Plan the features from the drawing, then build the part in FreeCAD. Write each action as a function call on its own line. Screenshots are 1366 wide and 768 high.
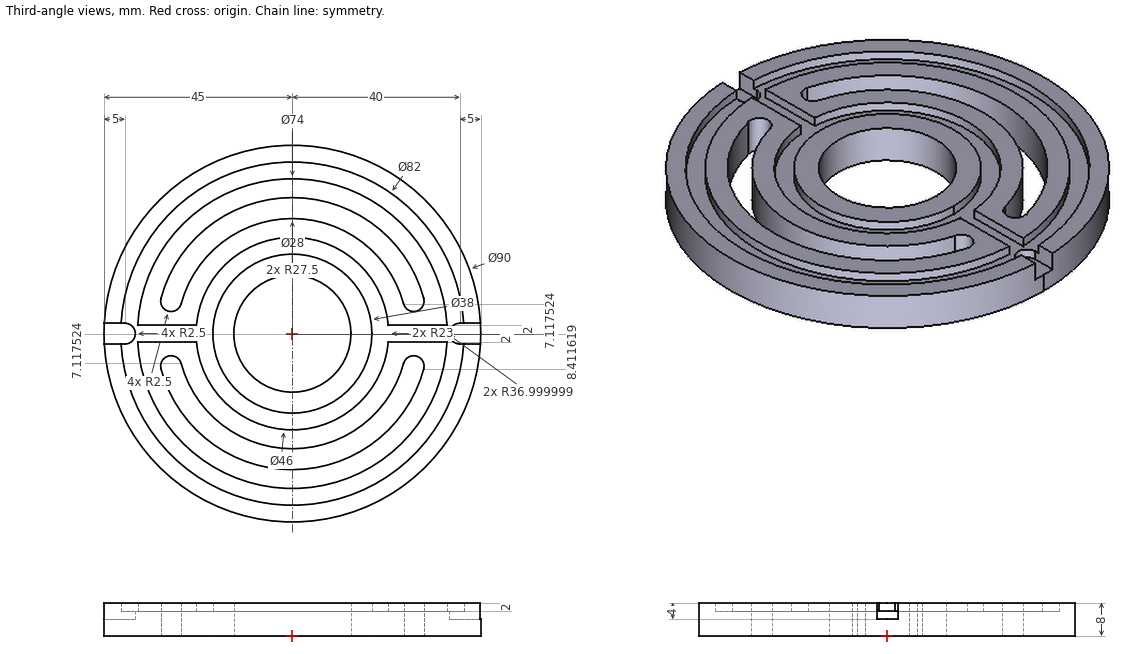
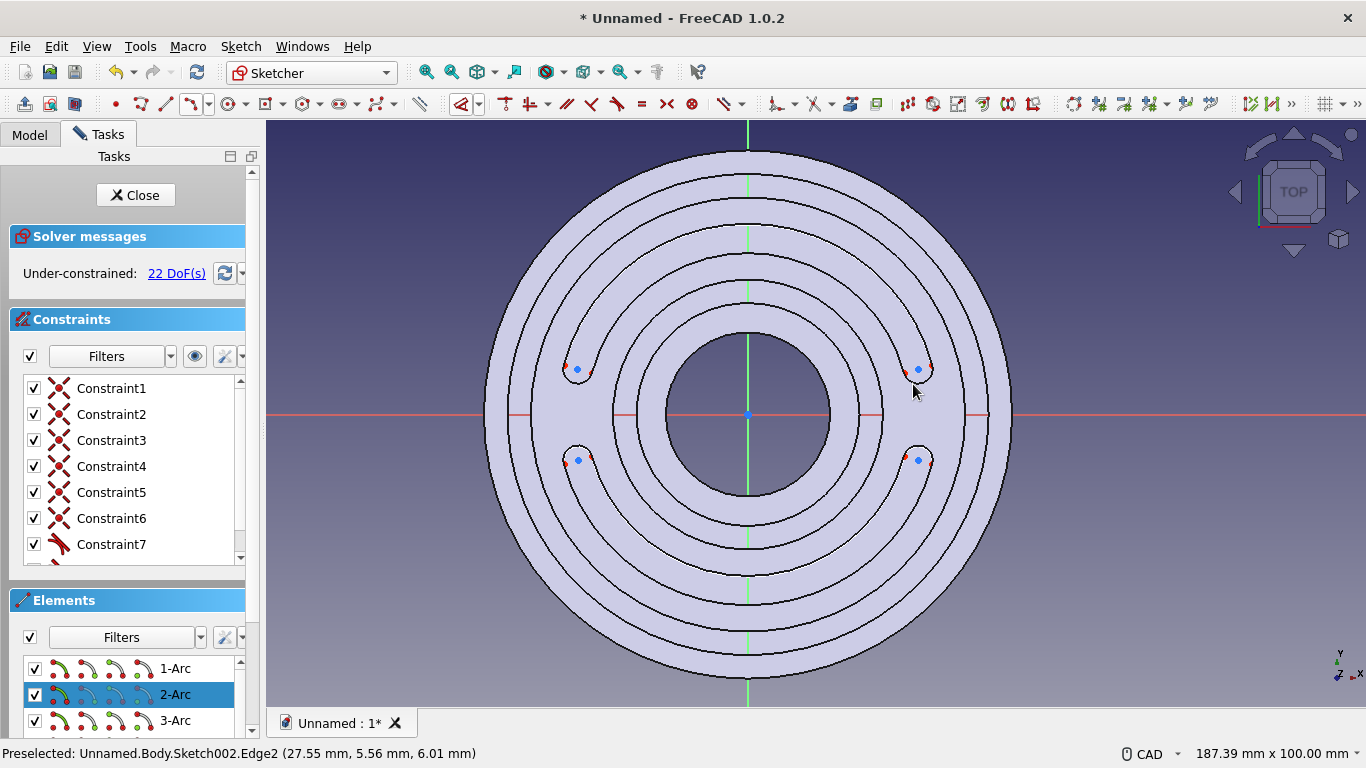
click(843, 250)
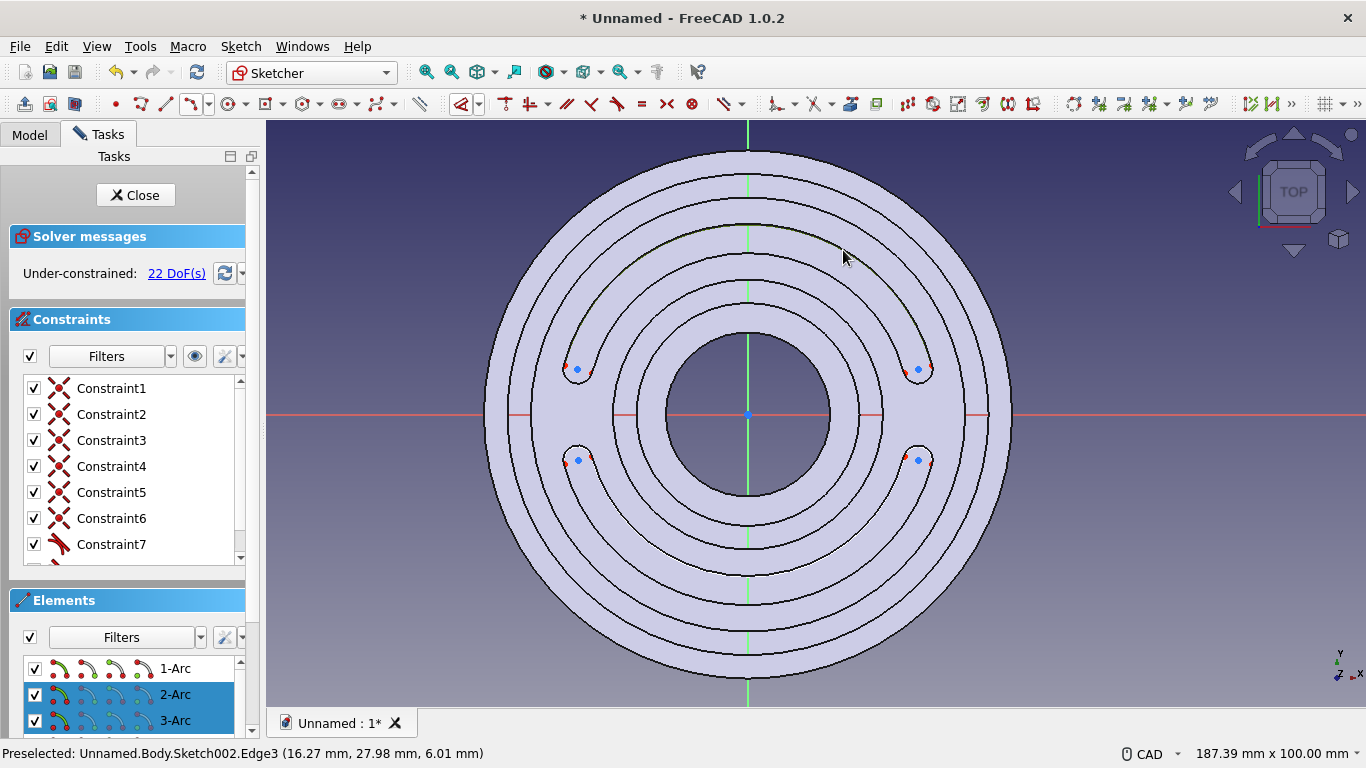
click(617, 104)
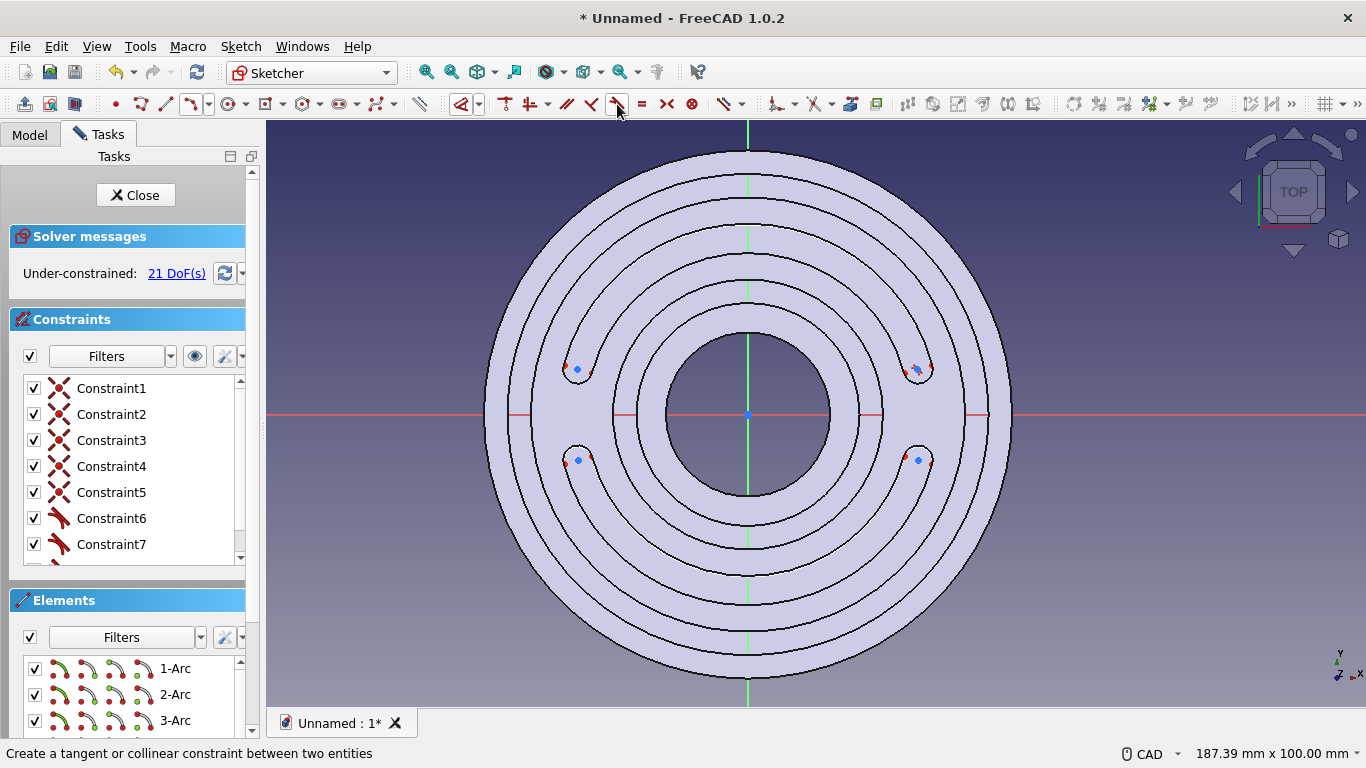
click(843, 250)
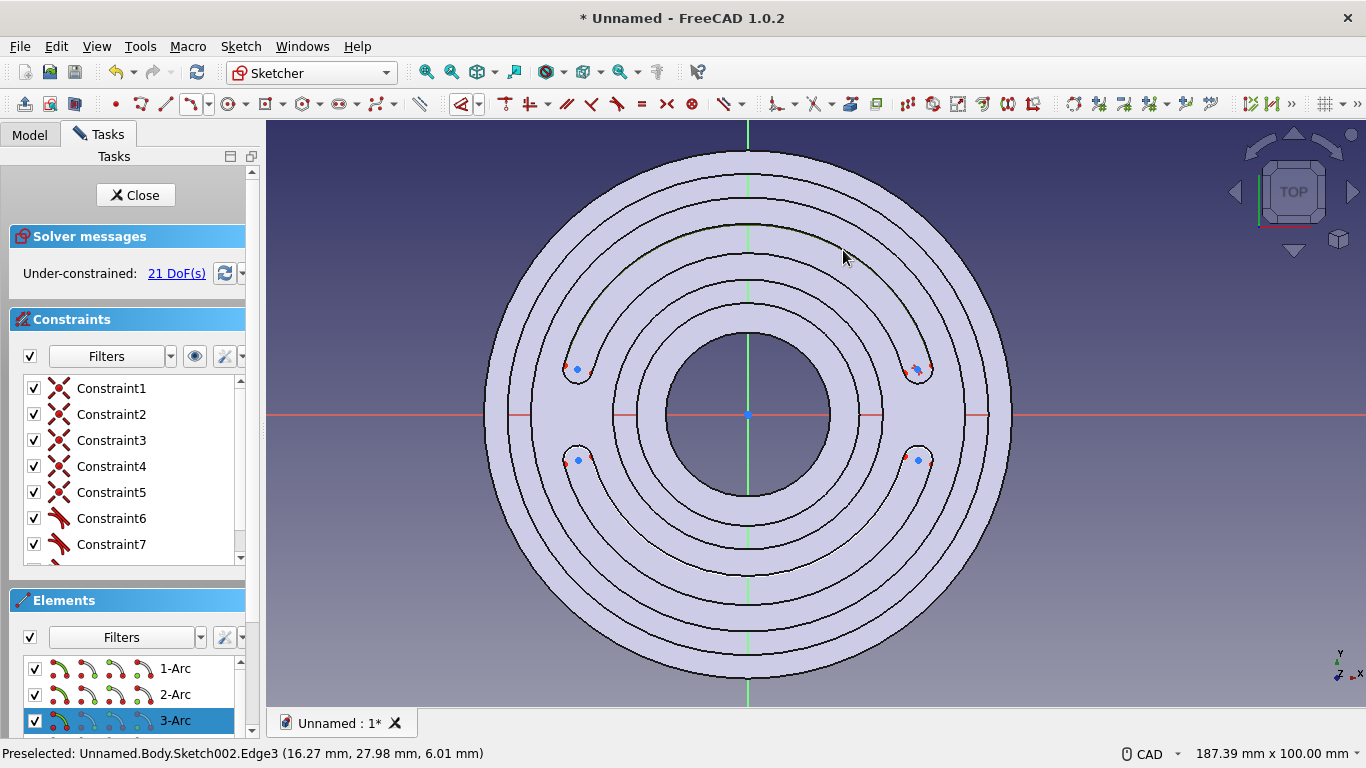
click(567, 379)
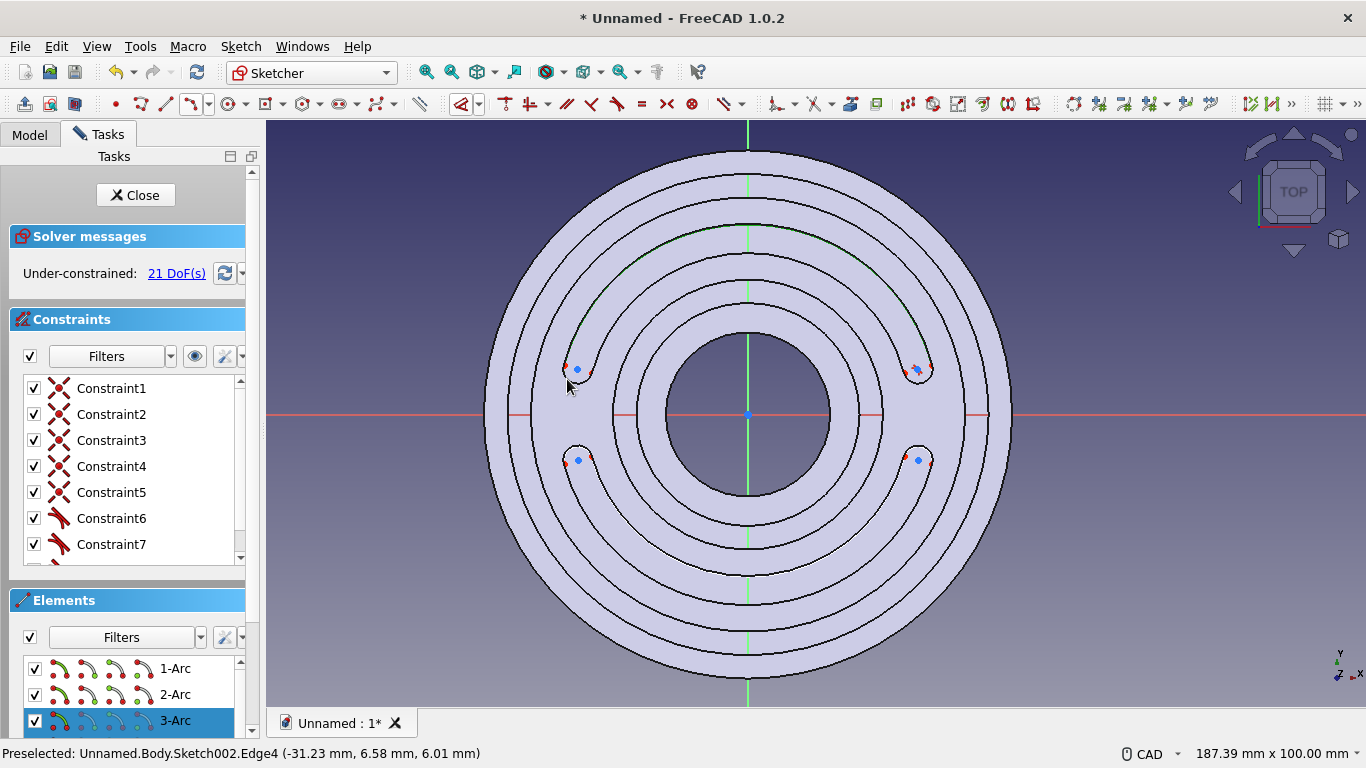
click(617, 104)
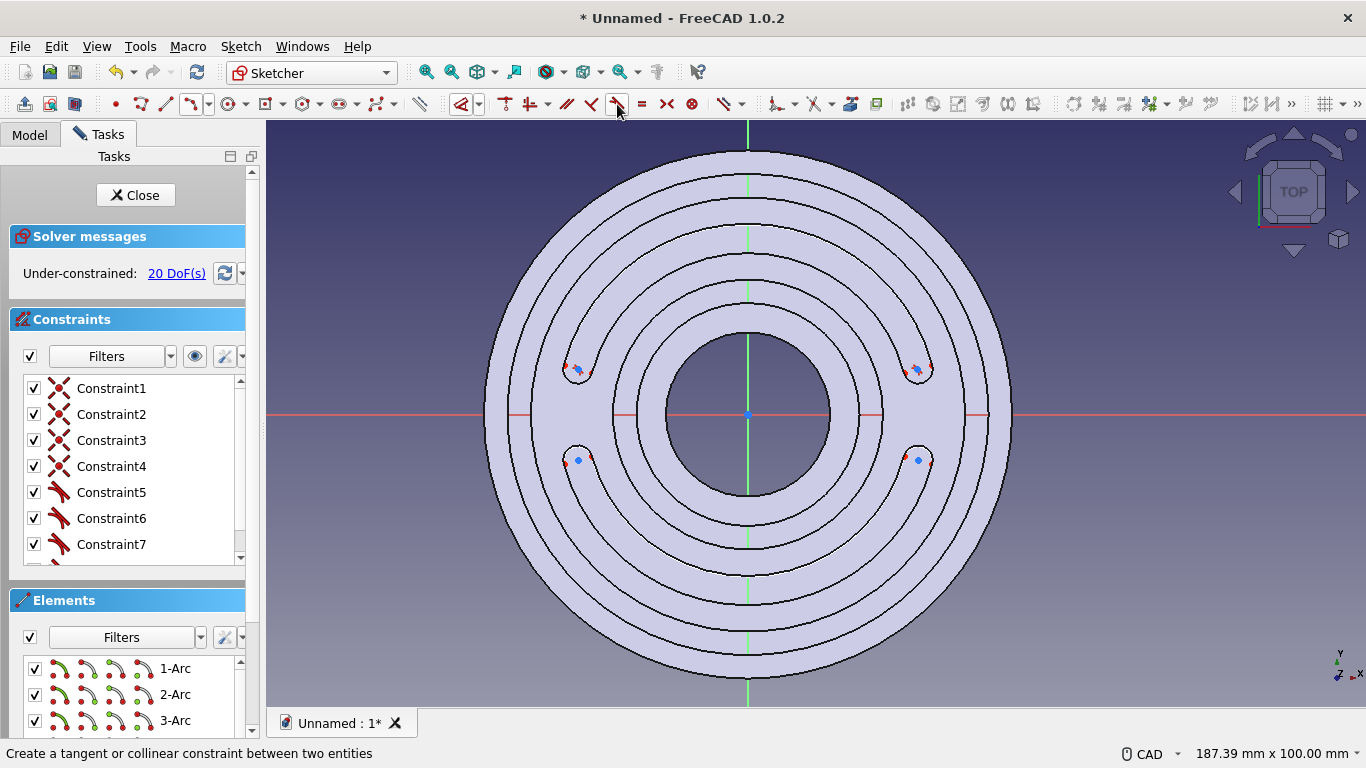
click(583, 447)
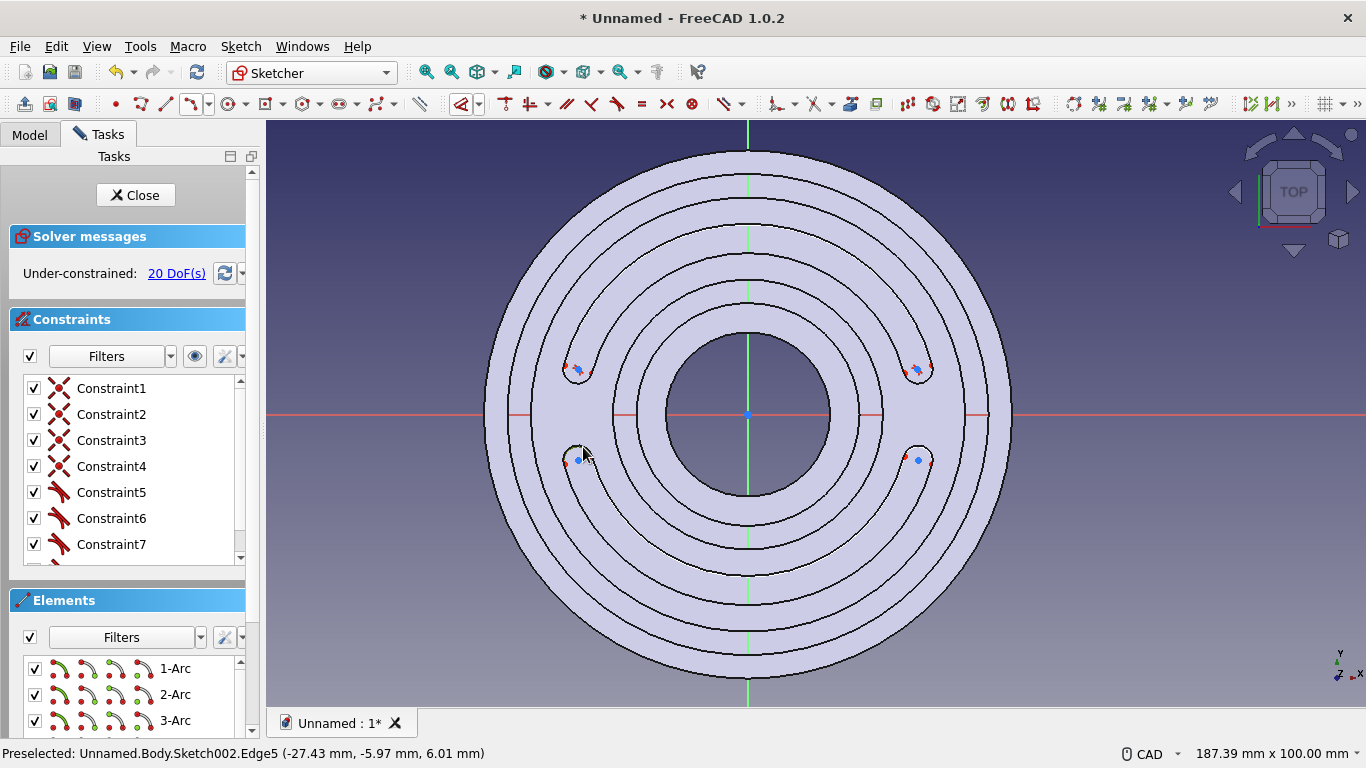
click(653, 581)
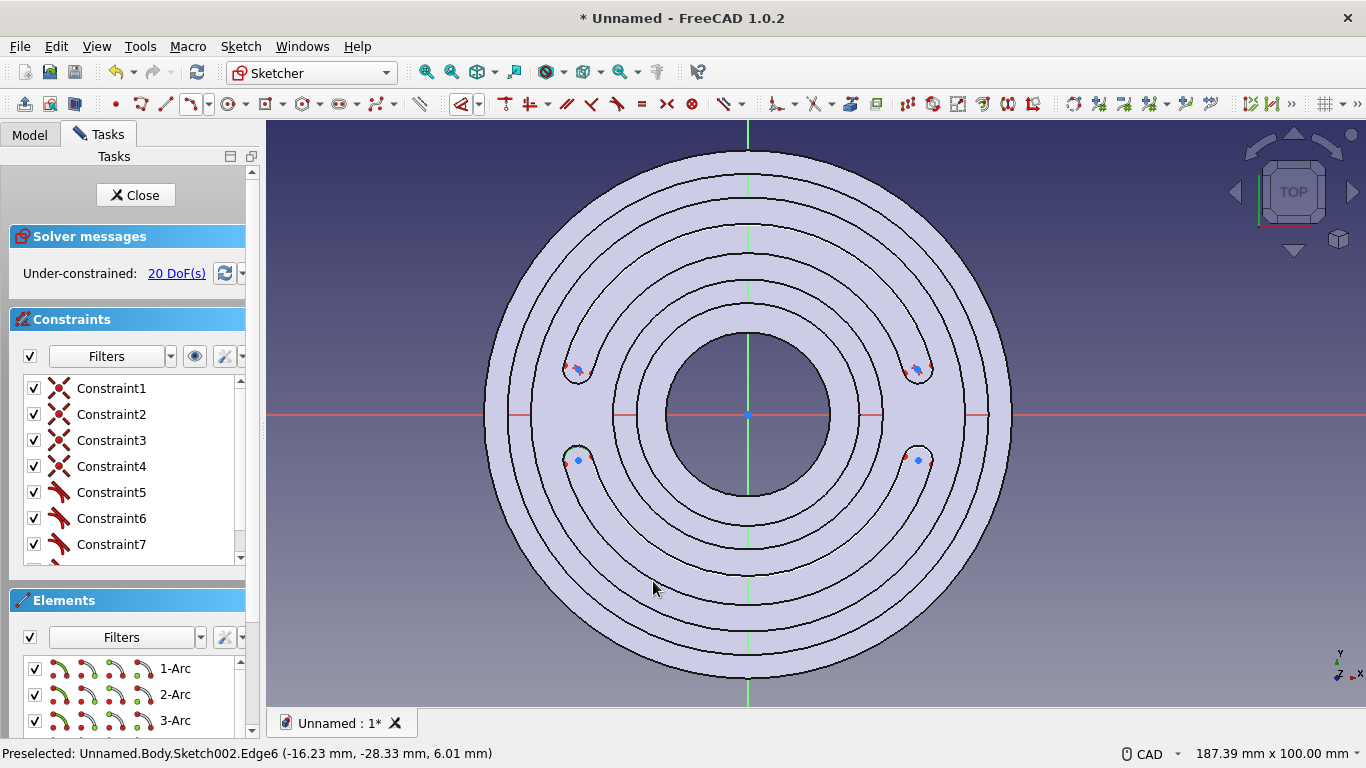
key(t)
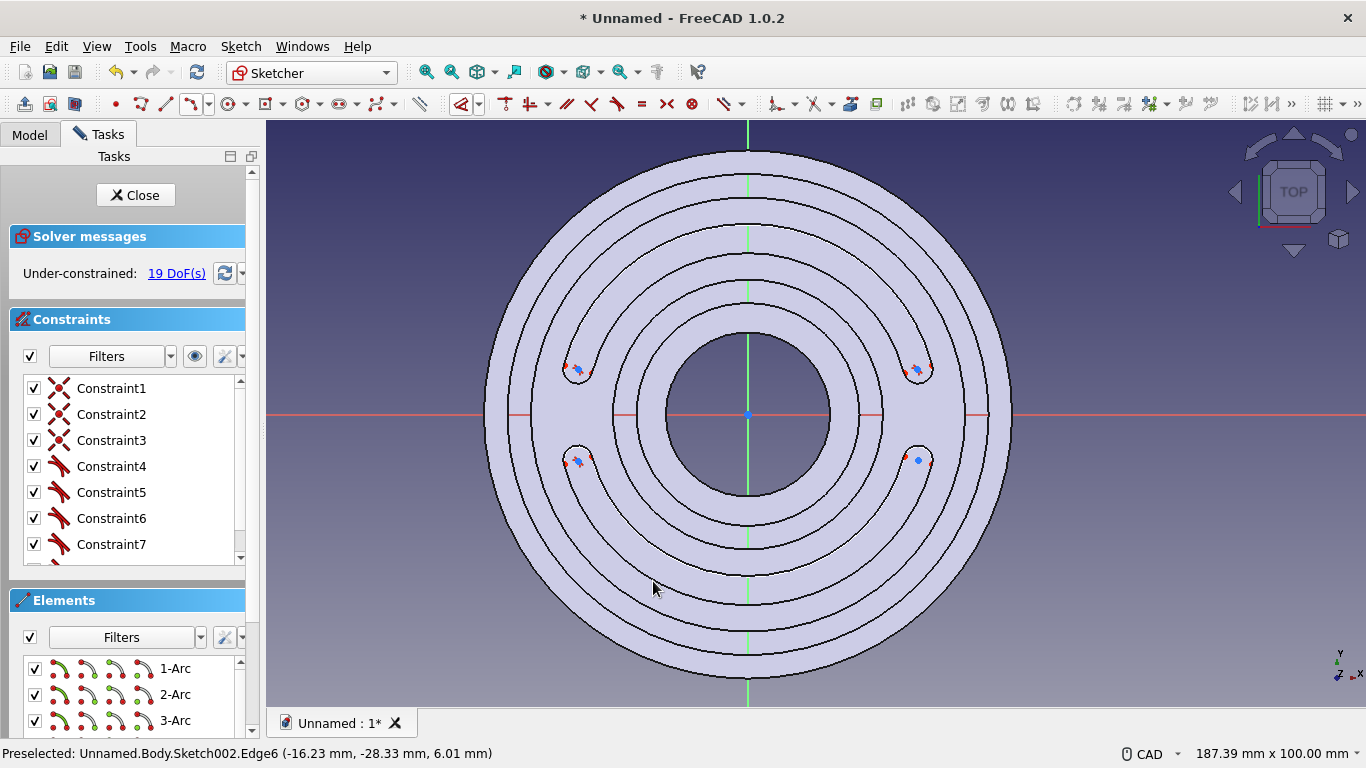
click(583, 448)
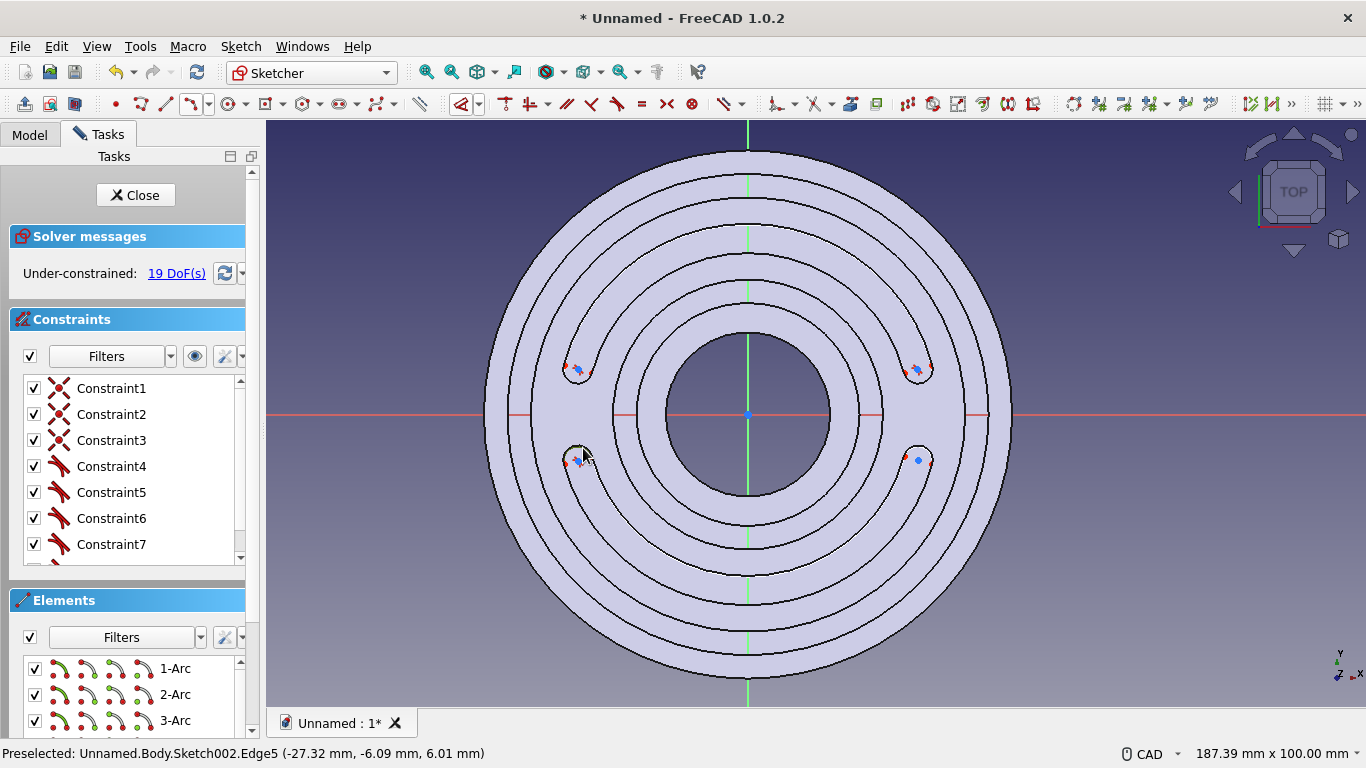
click(667, 555)